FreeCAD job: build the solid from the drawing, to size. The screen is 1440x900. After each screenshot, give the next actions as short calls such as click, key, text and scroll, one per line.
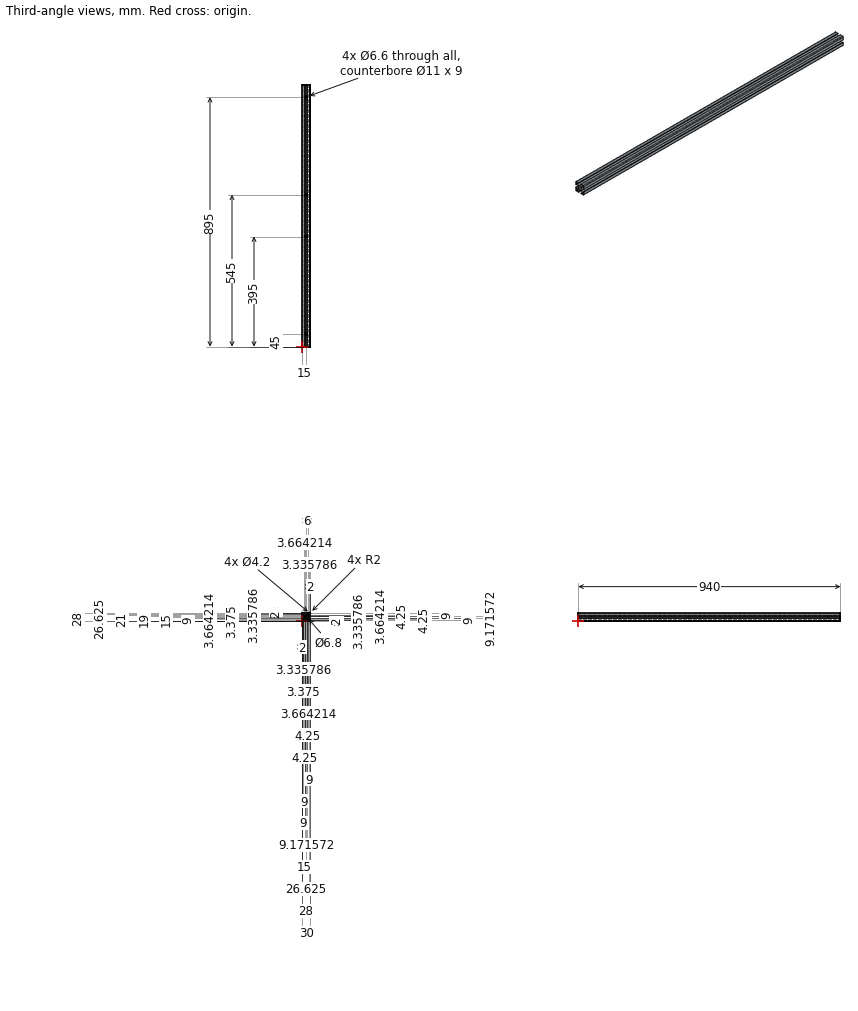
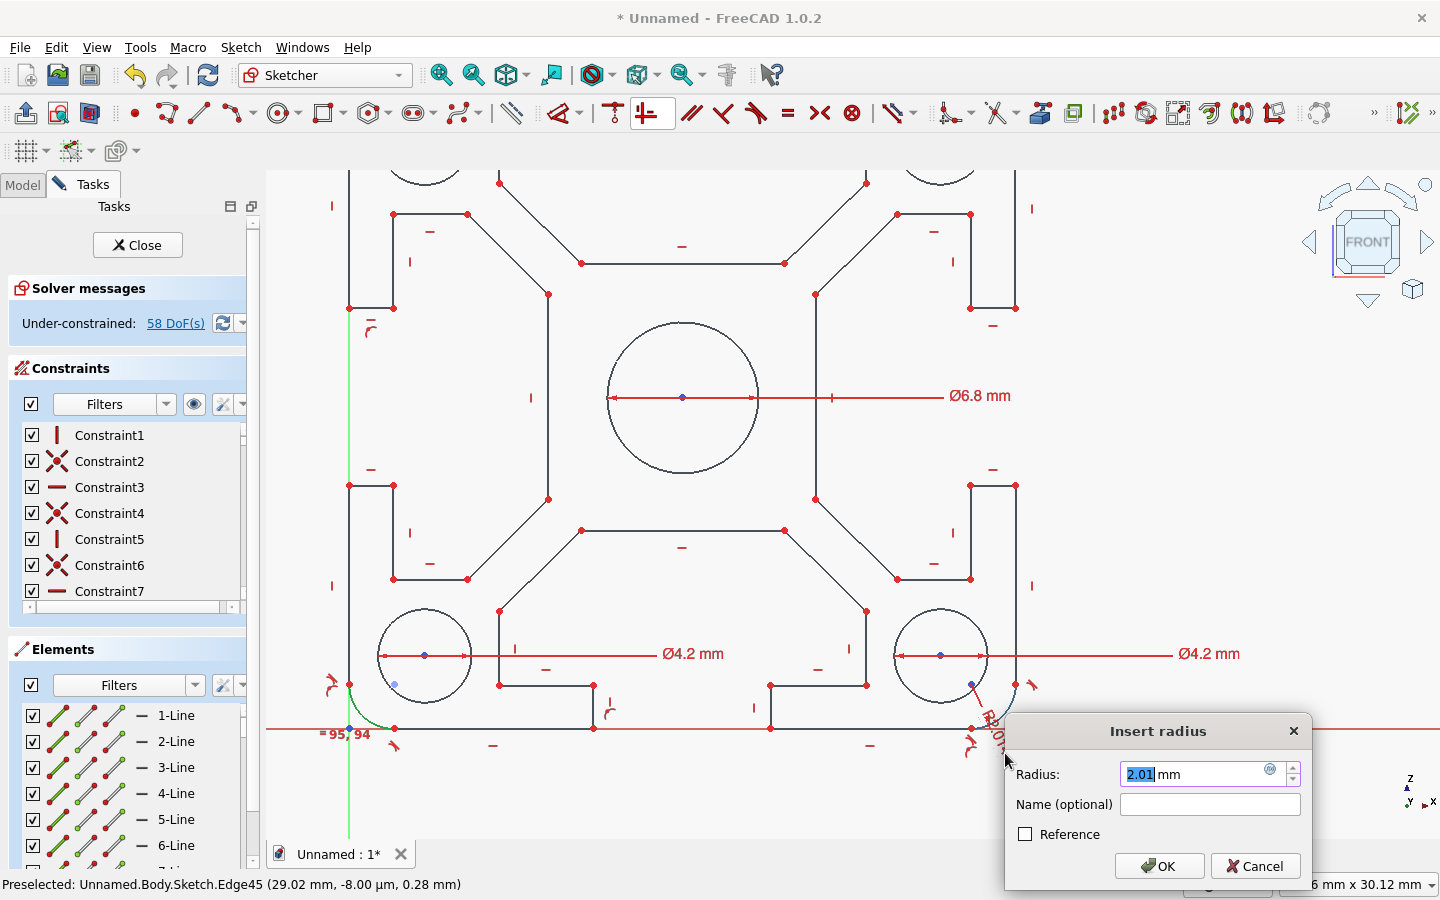
text(2)
key(Return)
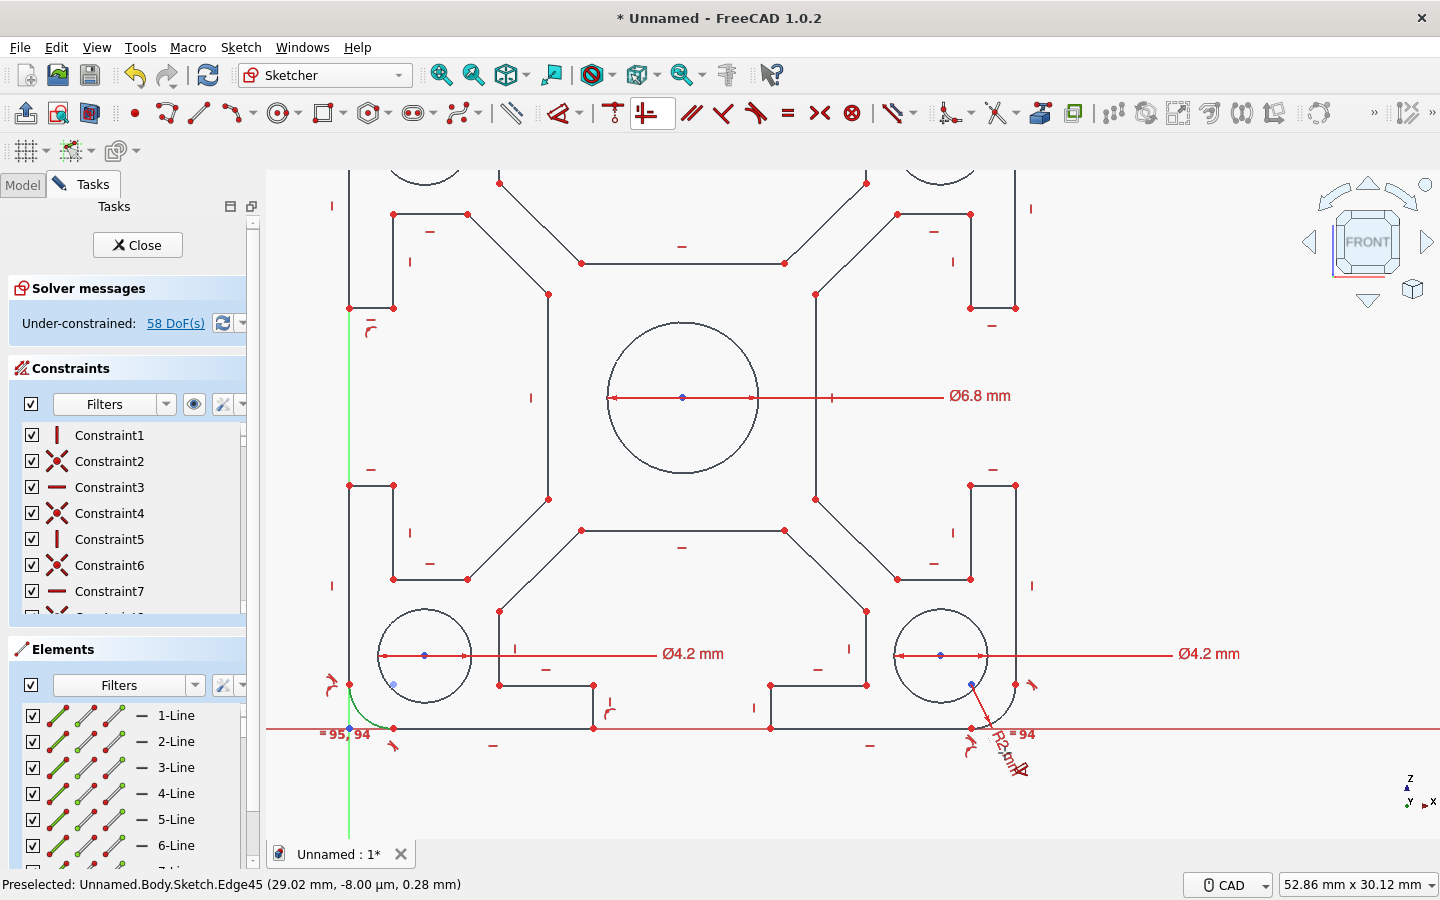
click(1015, 248)
click(1049, 253)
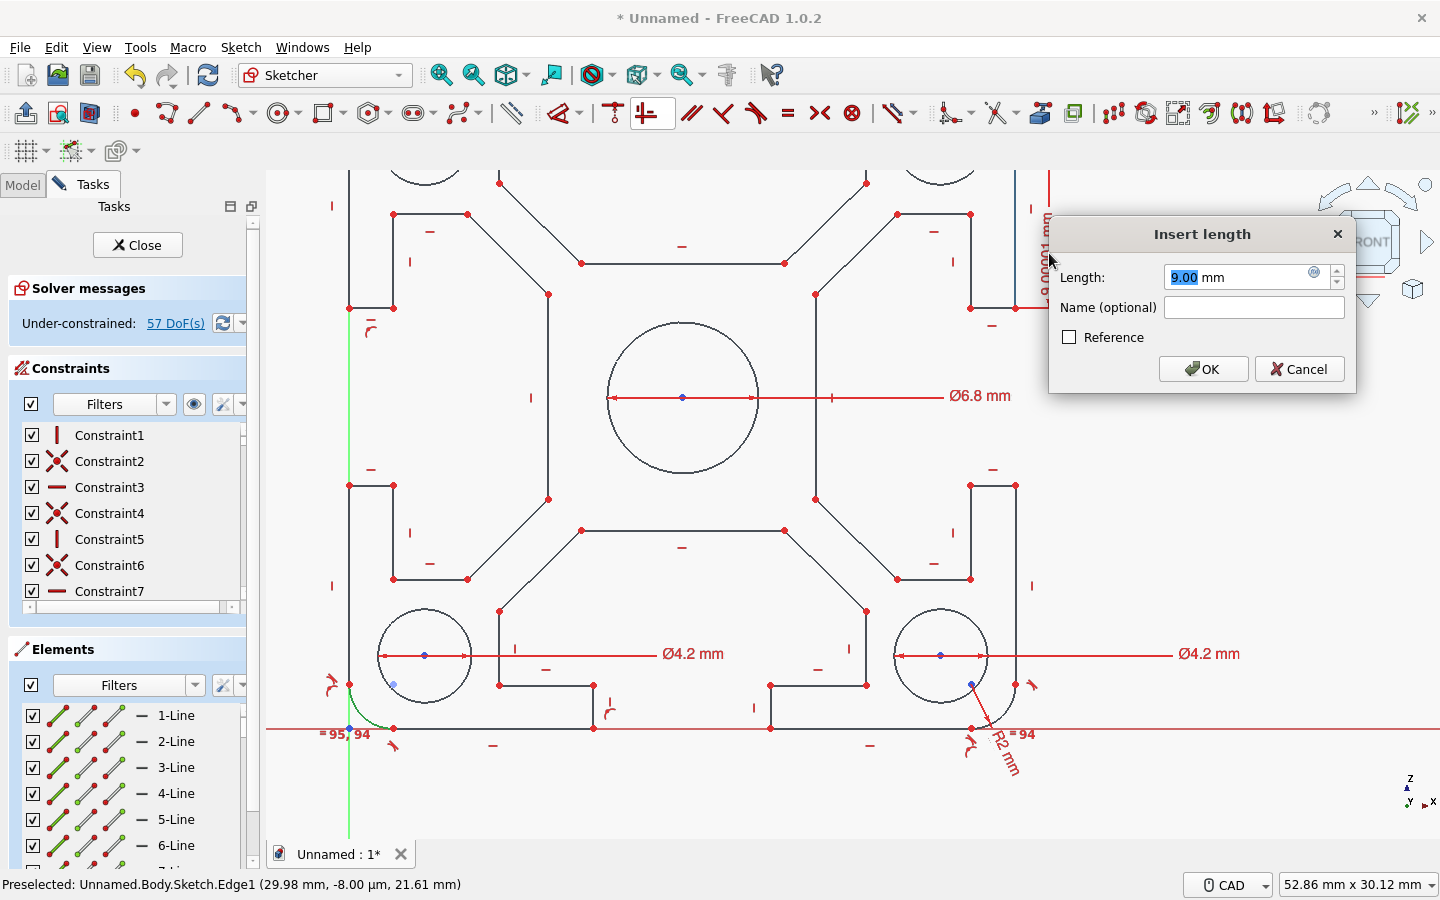
text(9)
key(Return)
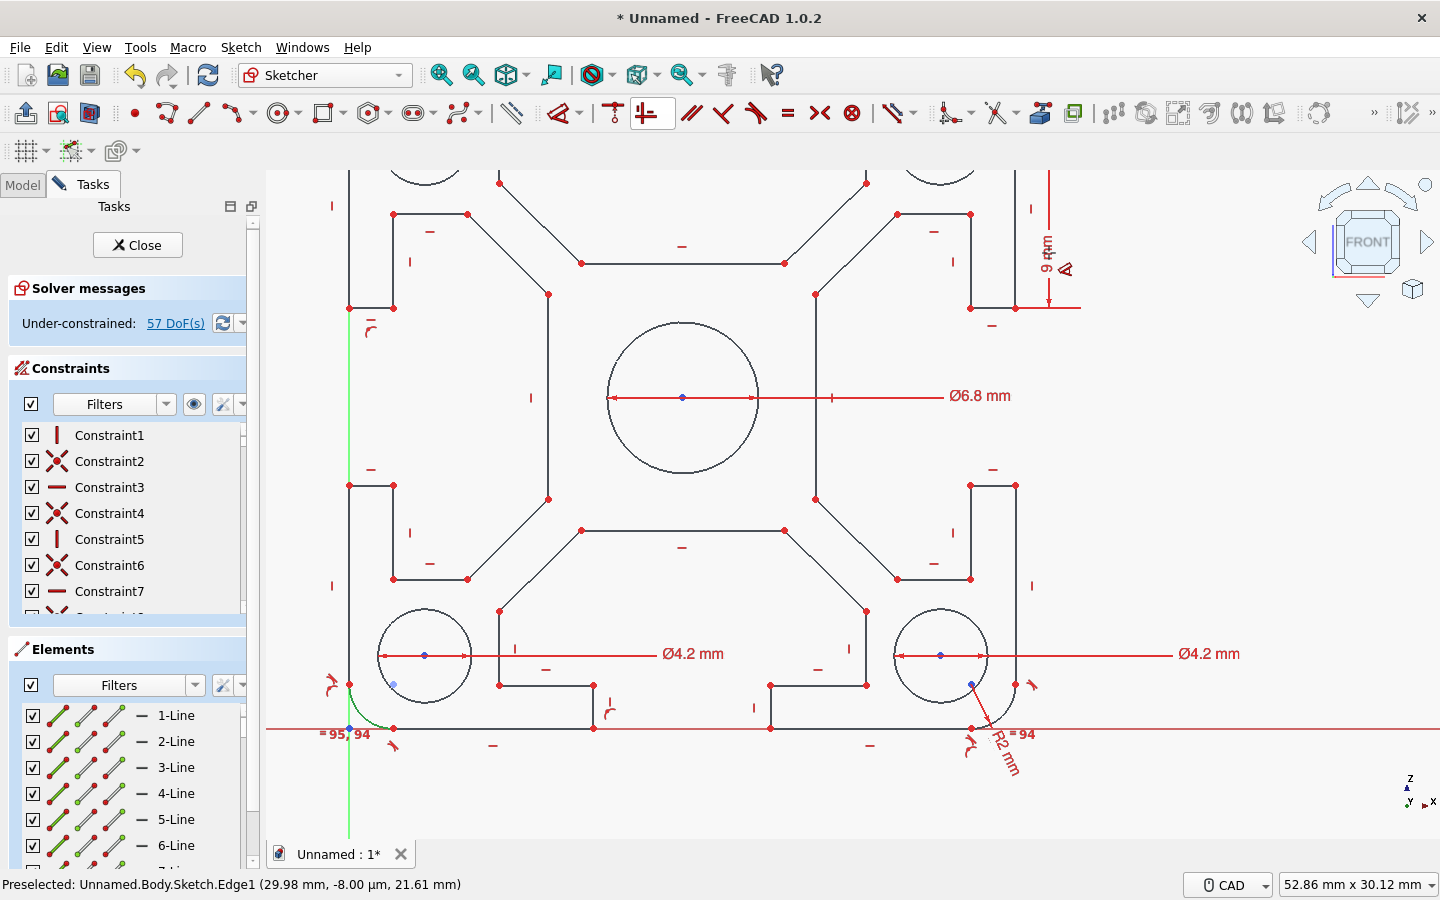
click(1002, 308)
click(993, 274)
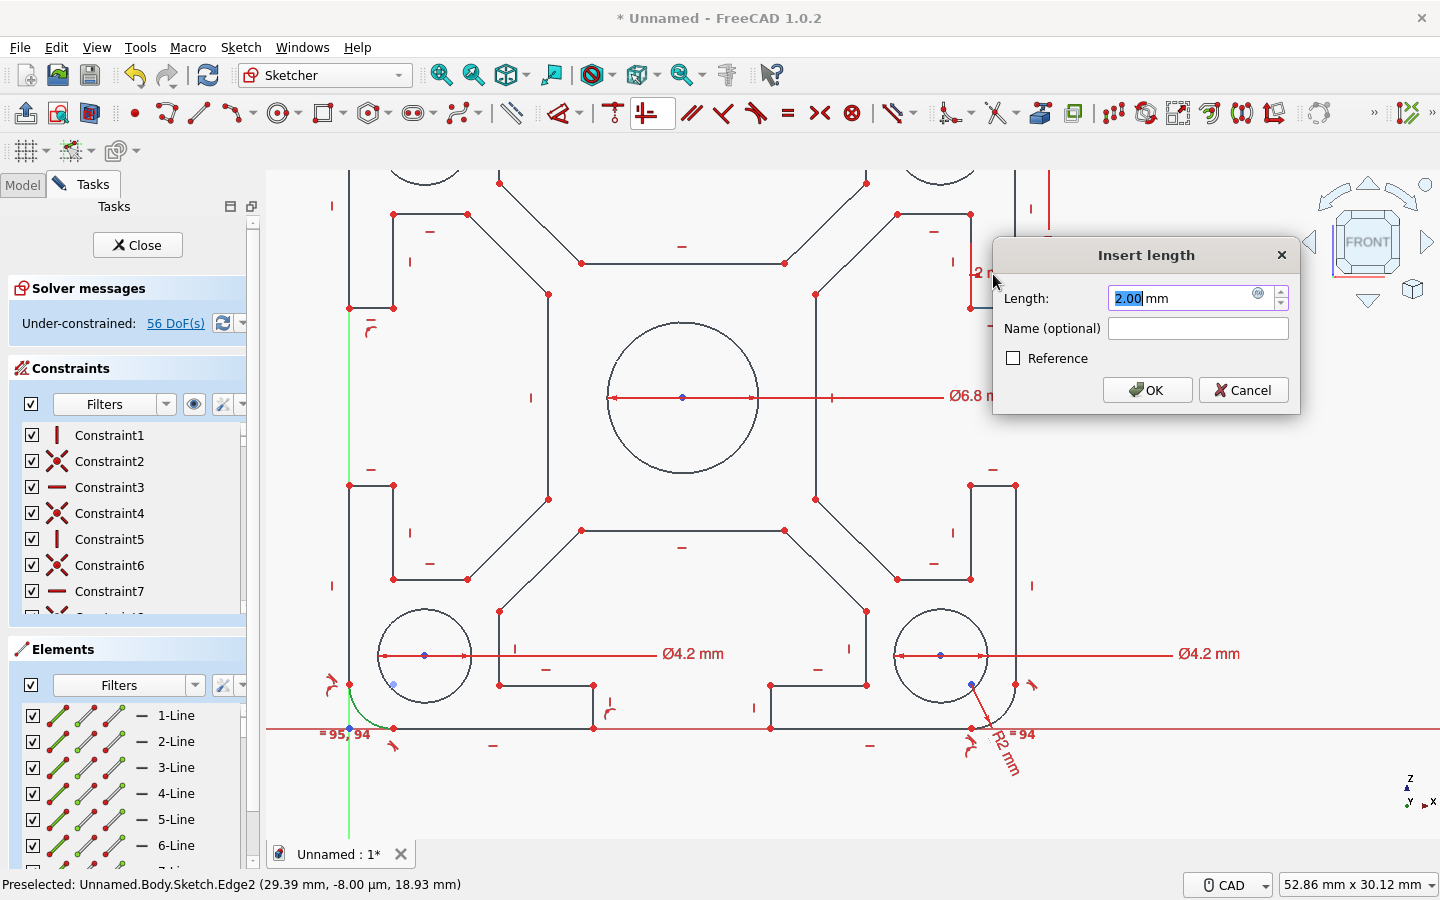
text(2)
key(Return)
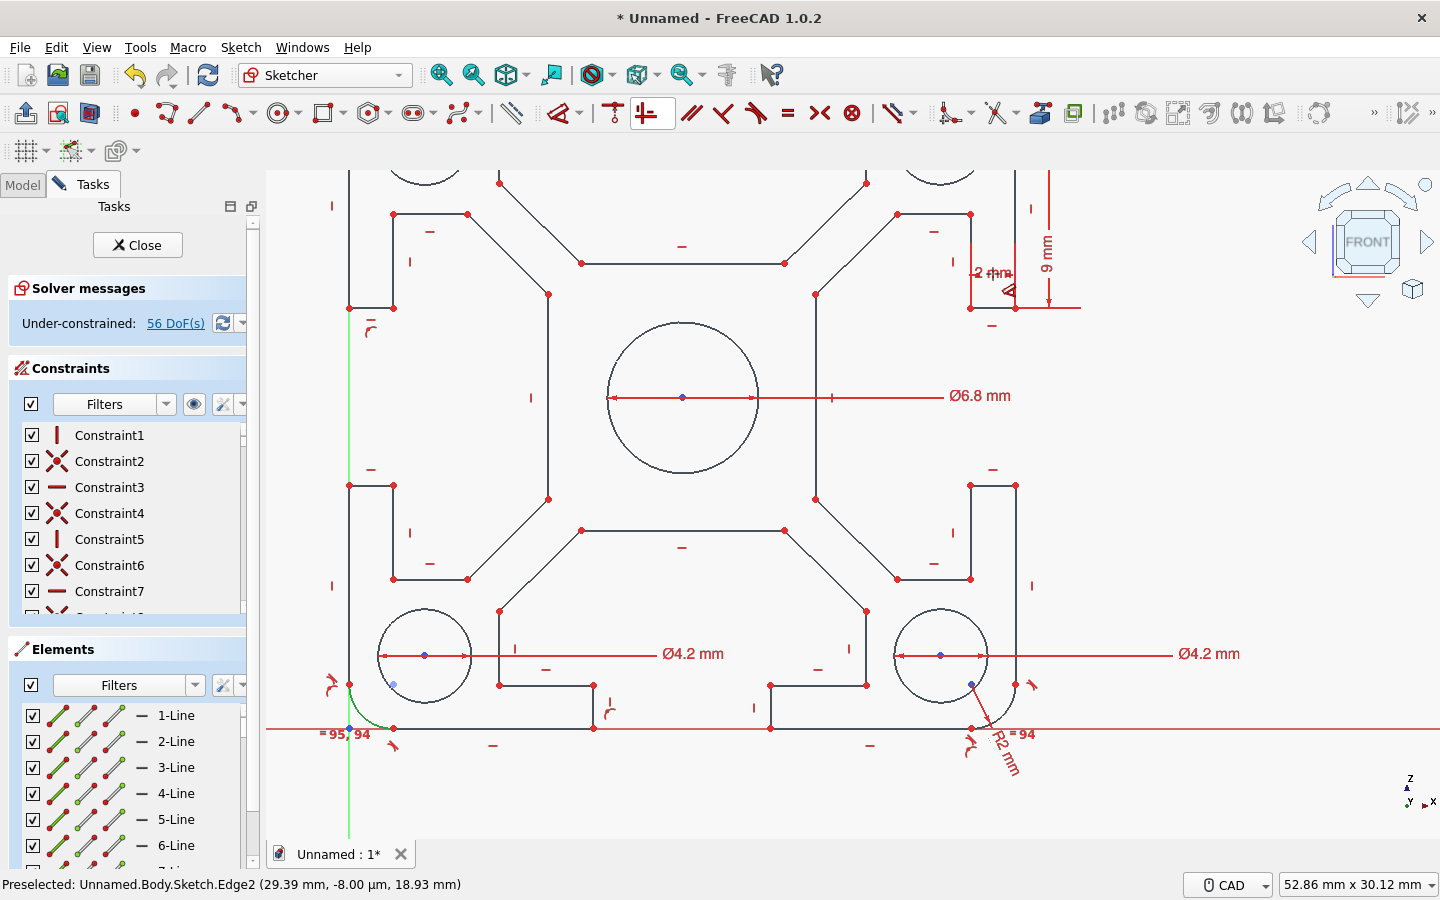
click(984, 486)
click(993, 520)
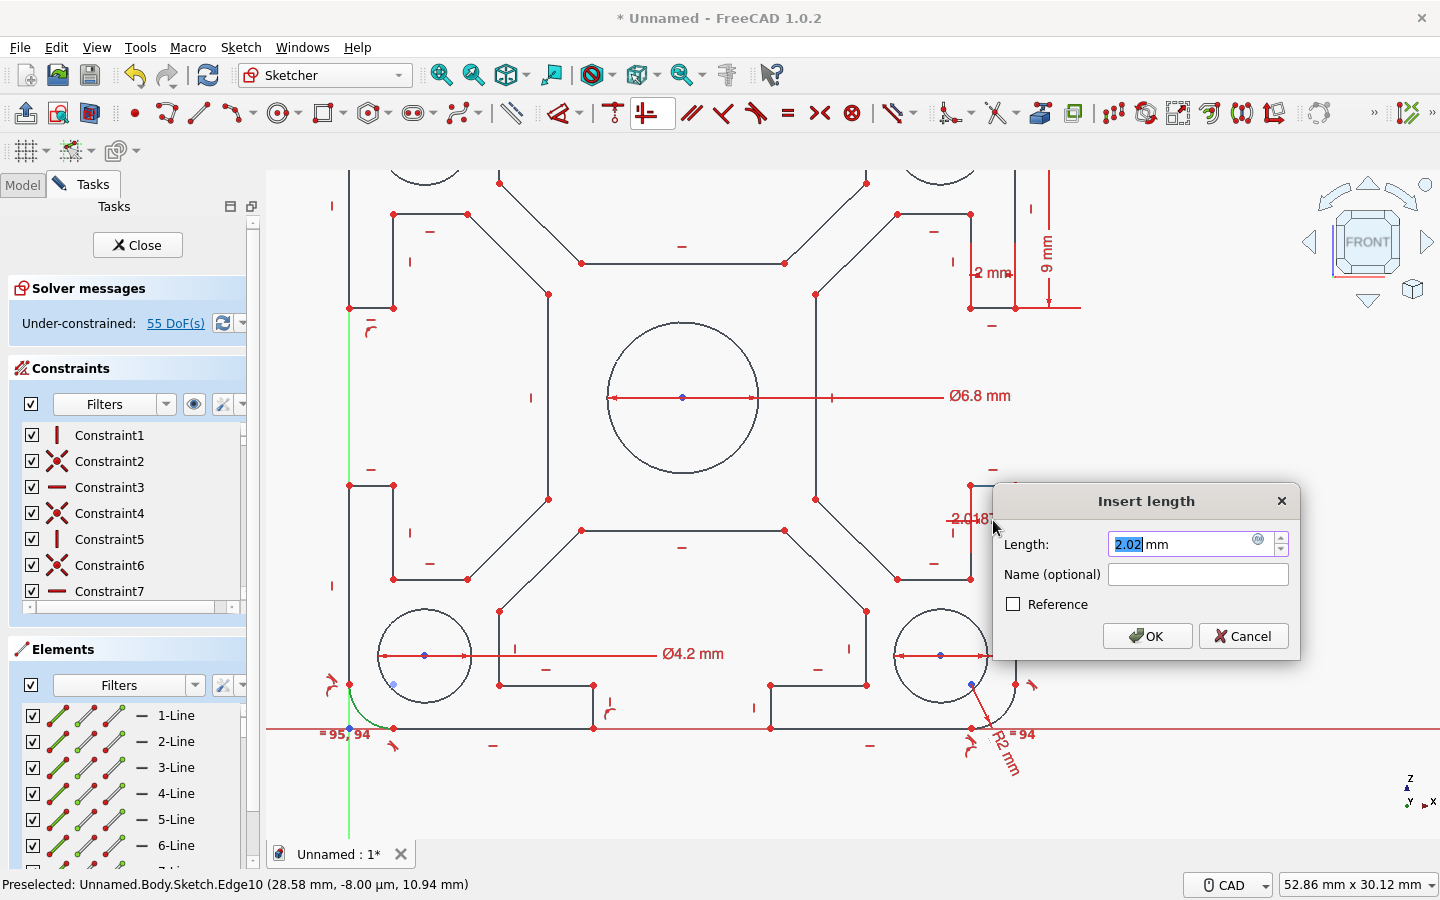
text(2)
key(Return)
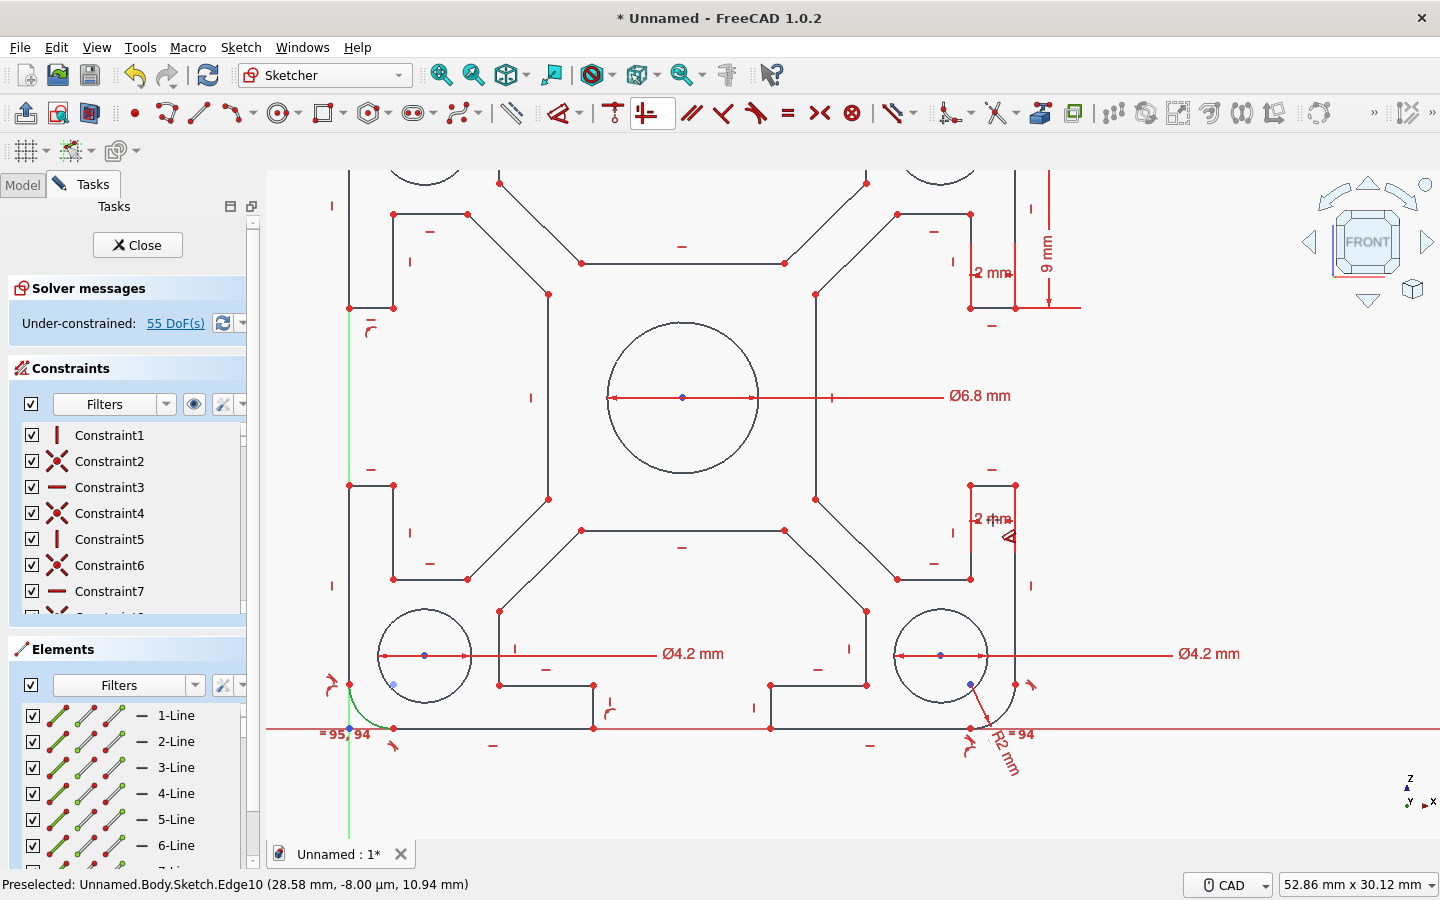
click(1015, 545)
click(1049, 585)